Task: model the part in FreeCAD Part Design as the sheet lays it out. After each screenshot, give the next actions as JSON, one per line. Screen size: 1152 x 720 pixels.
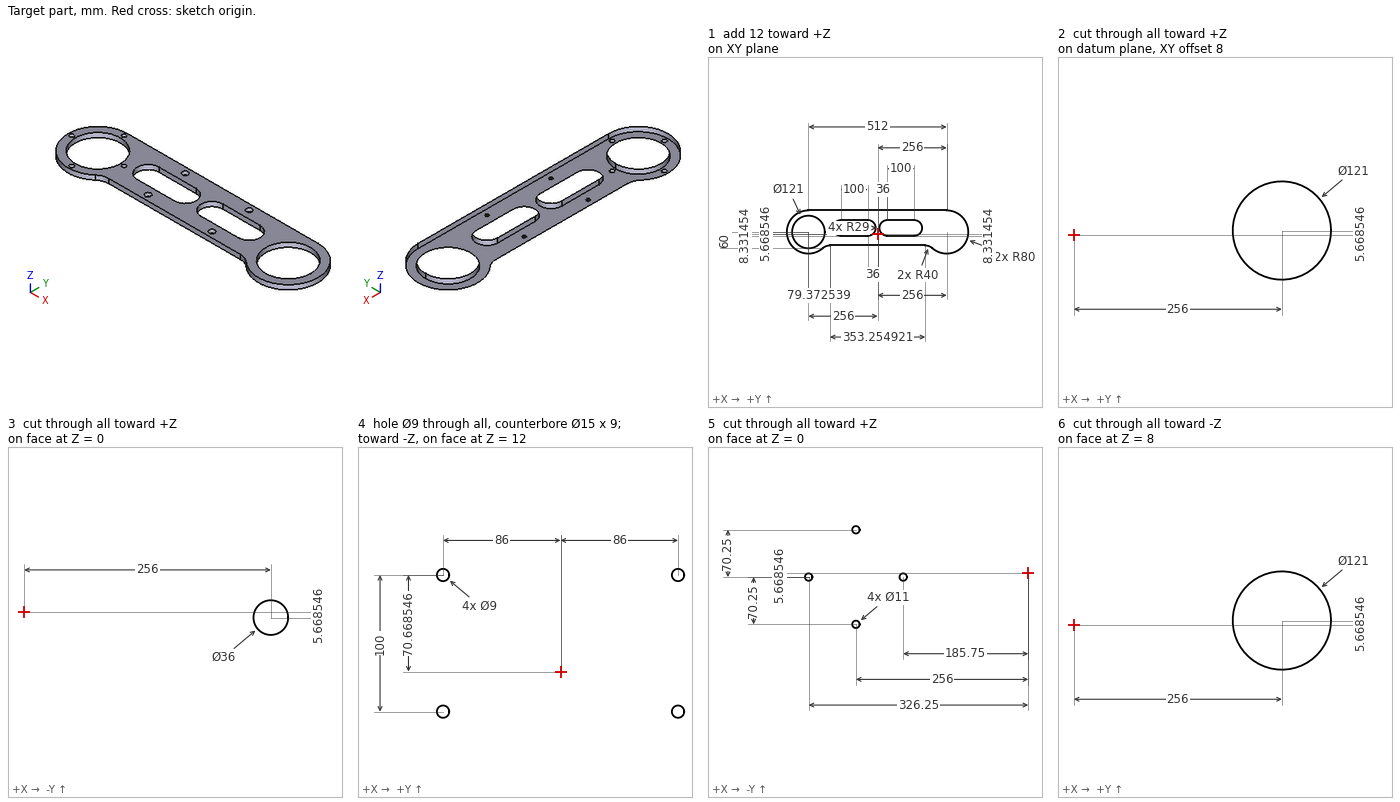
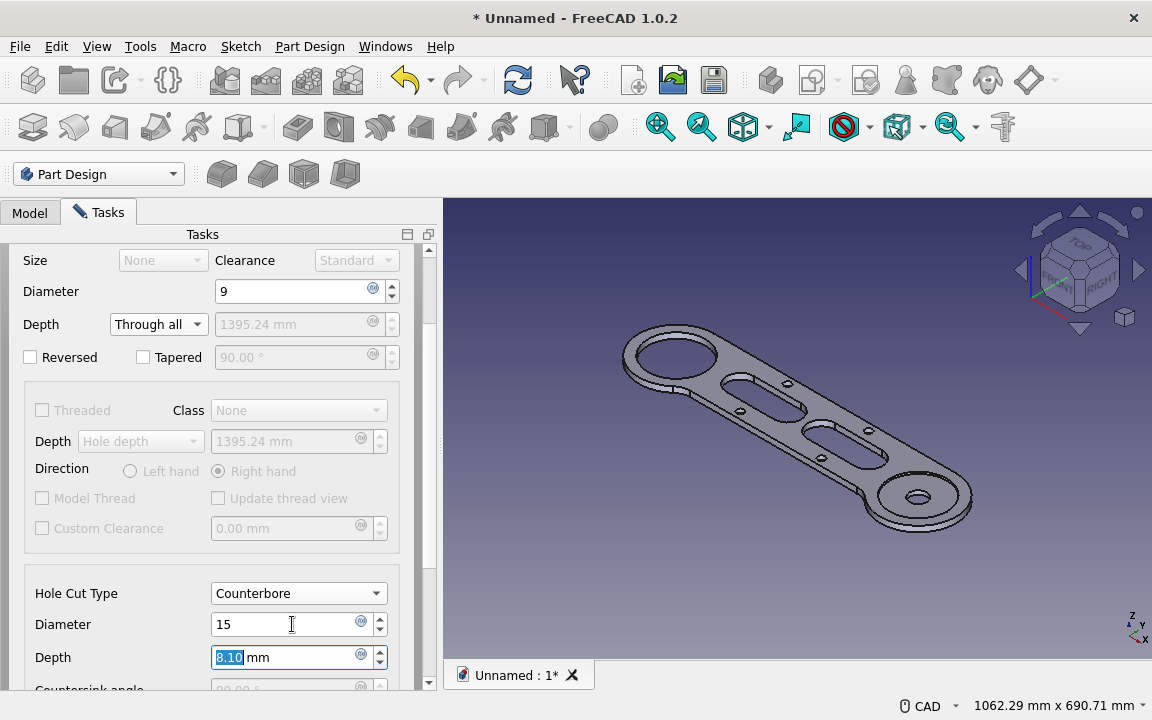
{"action": "type", "text": "9"}
{"action": "key", "text": "Tab"}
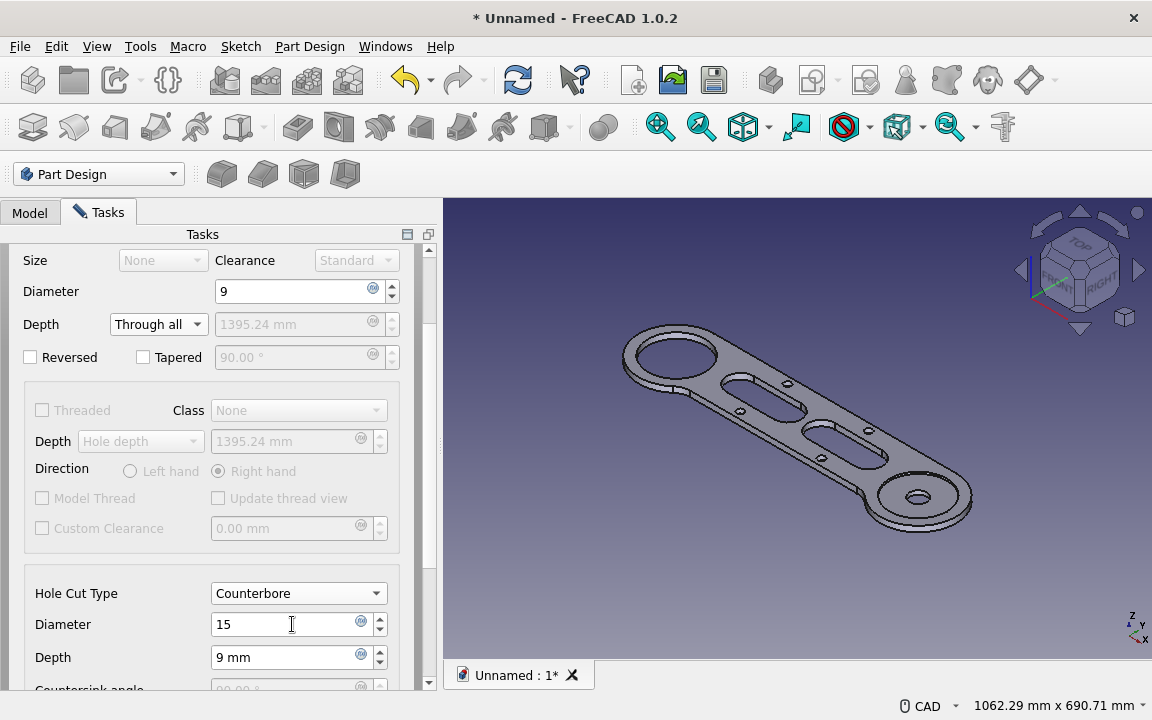
{"action": "scroll", "coordinate": [429, 467], "scroll_direction": "up", "scroll_amount": 3}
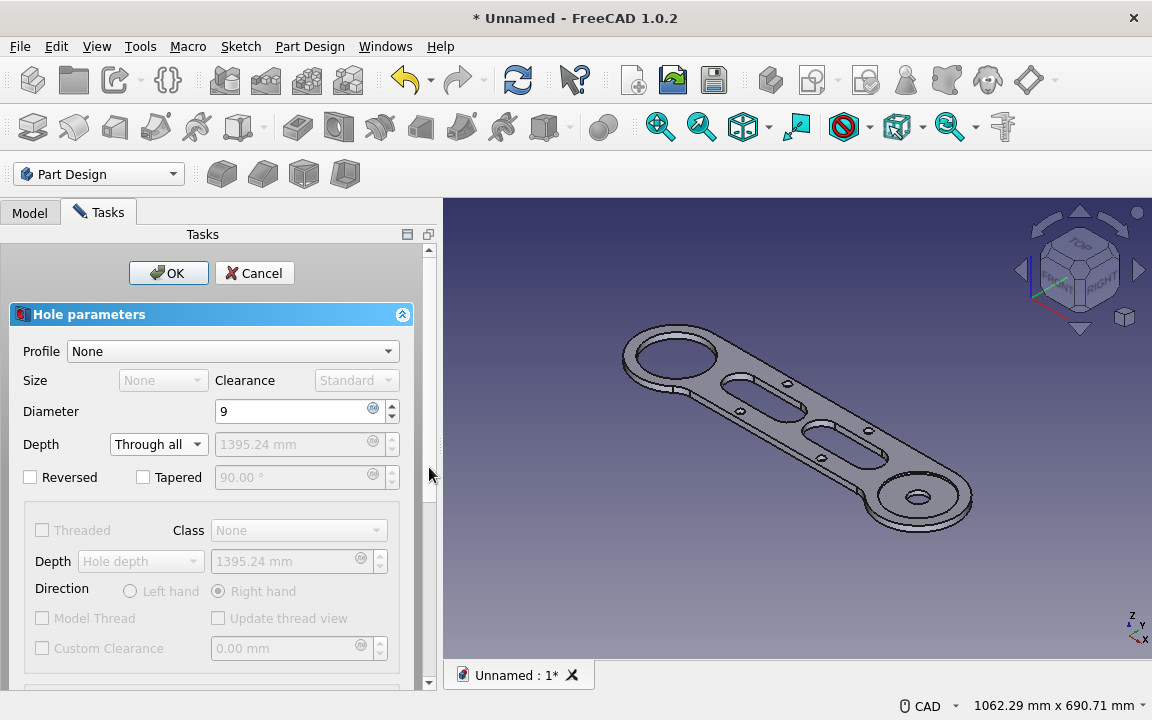
{"action": "left_click", "coordinate": [169, 273]}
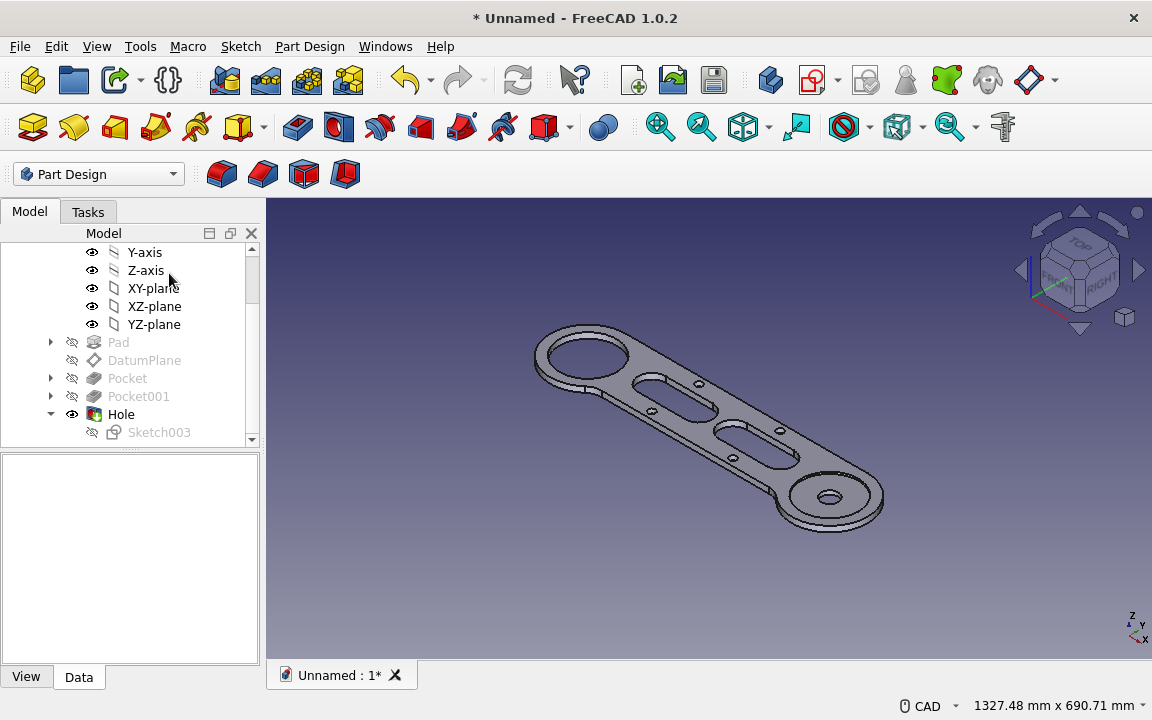
{"action": "key", "text": "5"}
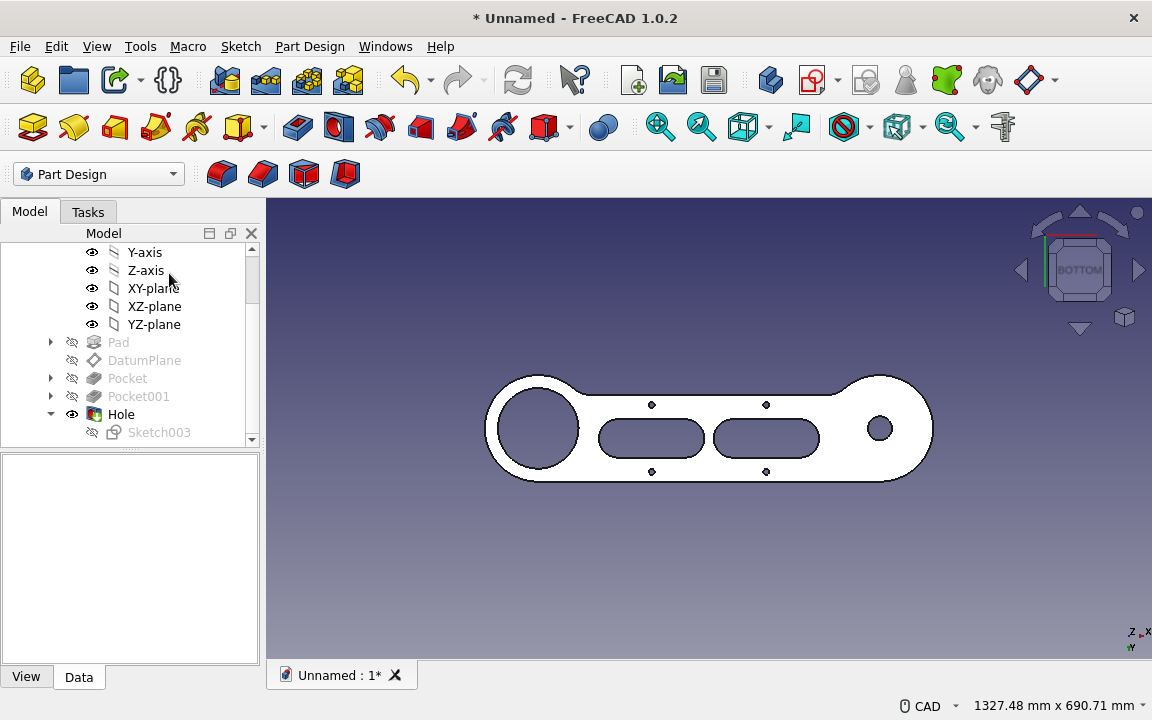
{"action": "left_click", "coordinate": [837, 458]}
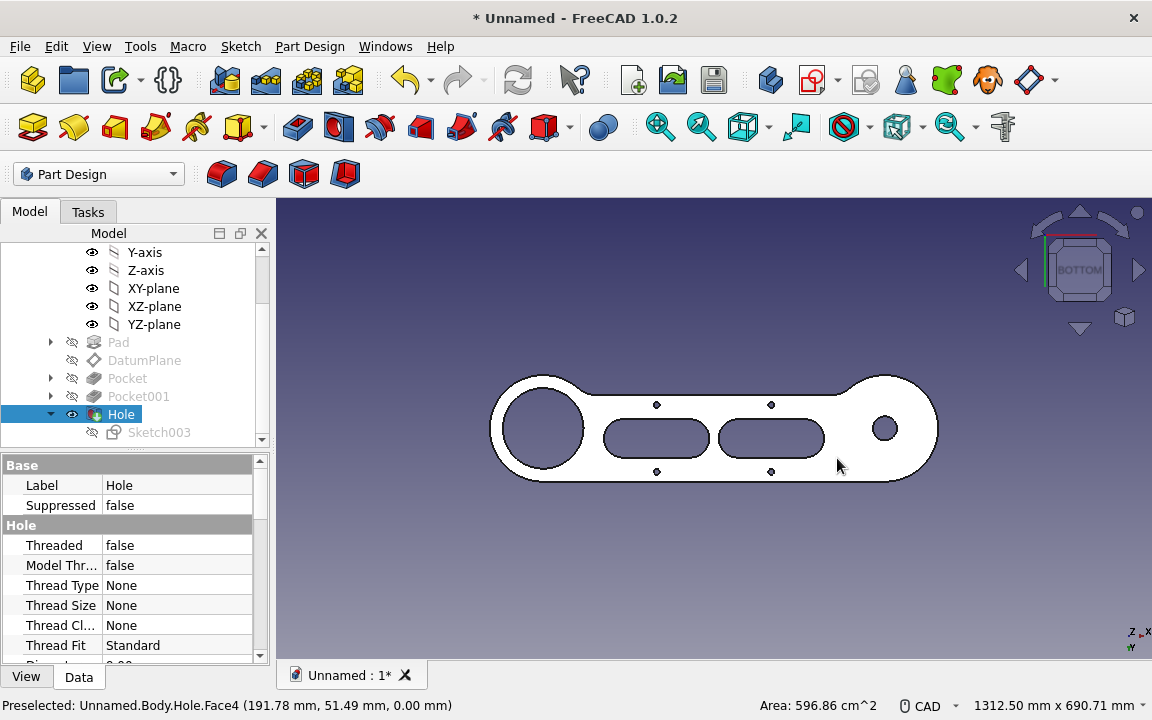
{"action": "left_click", "coordinate": [812, 80]}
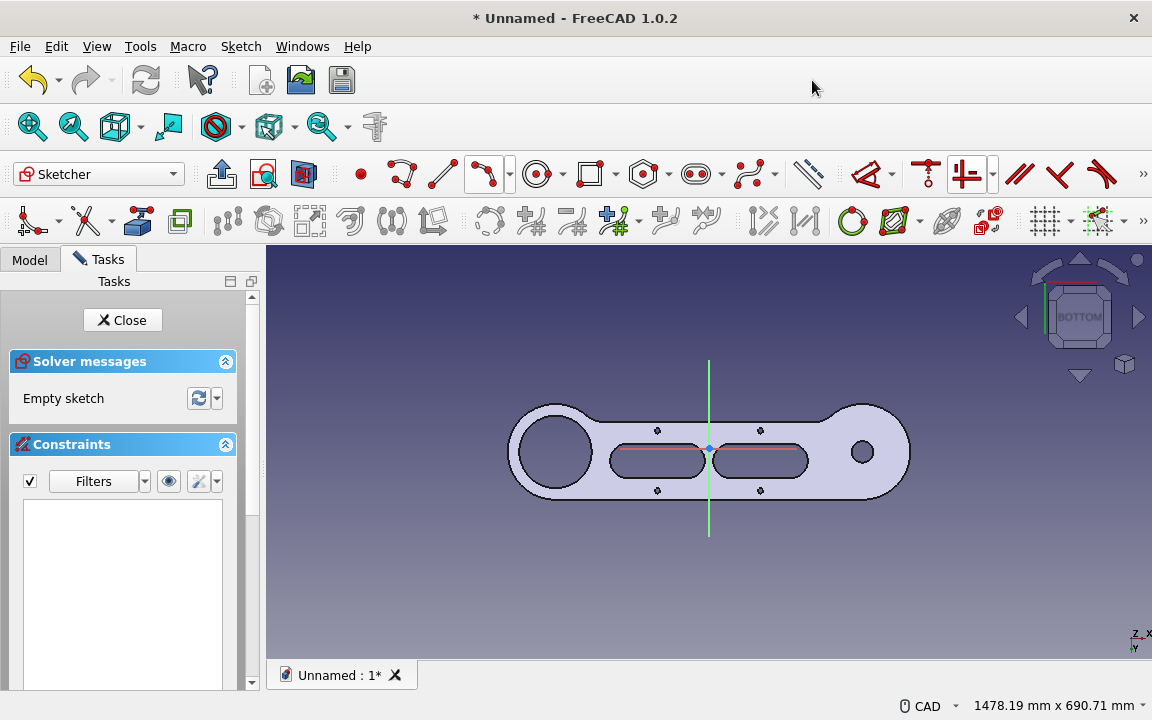
{"action": "scroll", "coordinate": [592, 452], "scroll_direction": "up", "scroll_amount": 5}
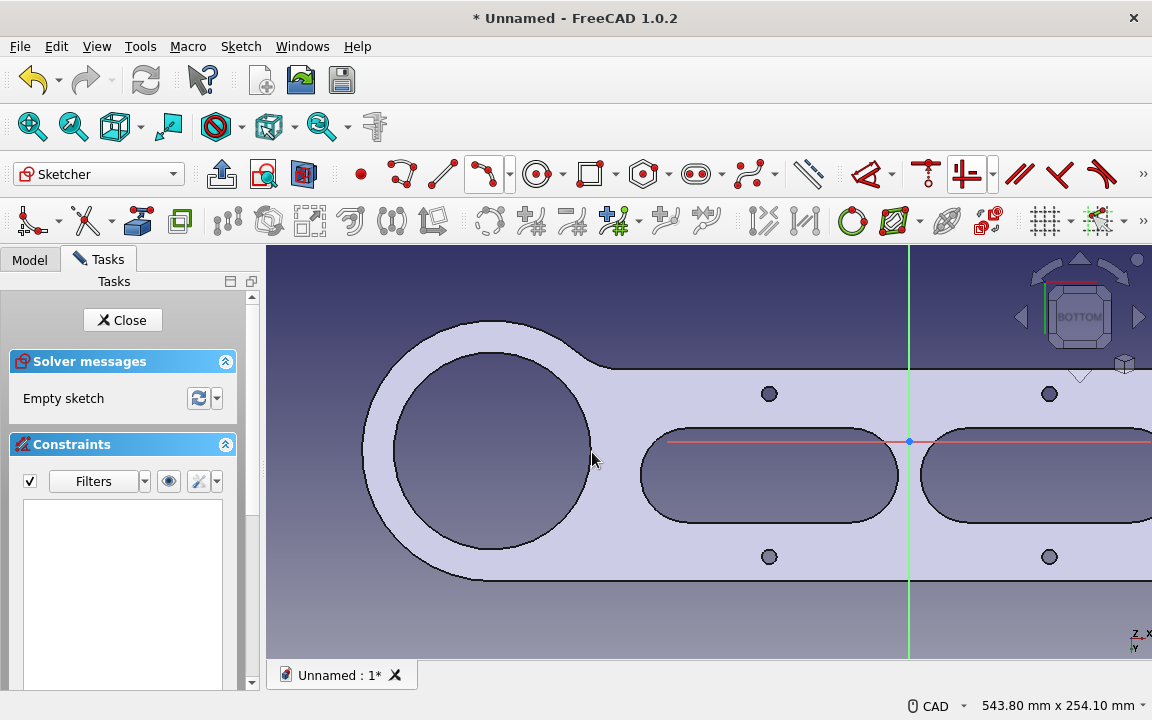
{"action": "left_click", "coordinate": [536, 174]}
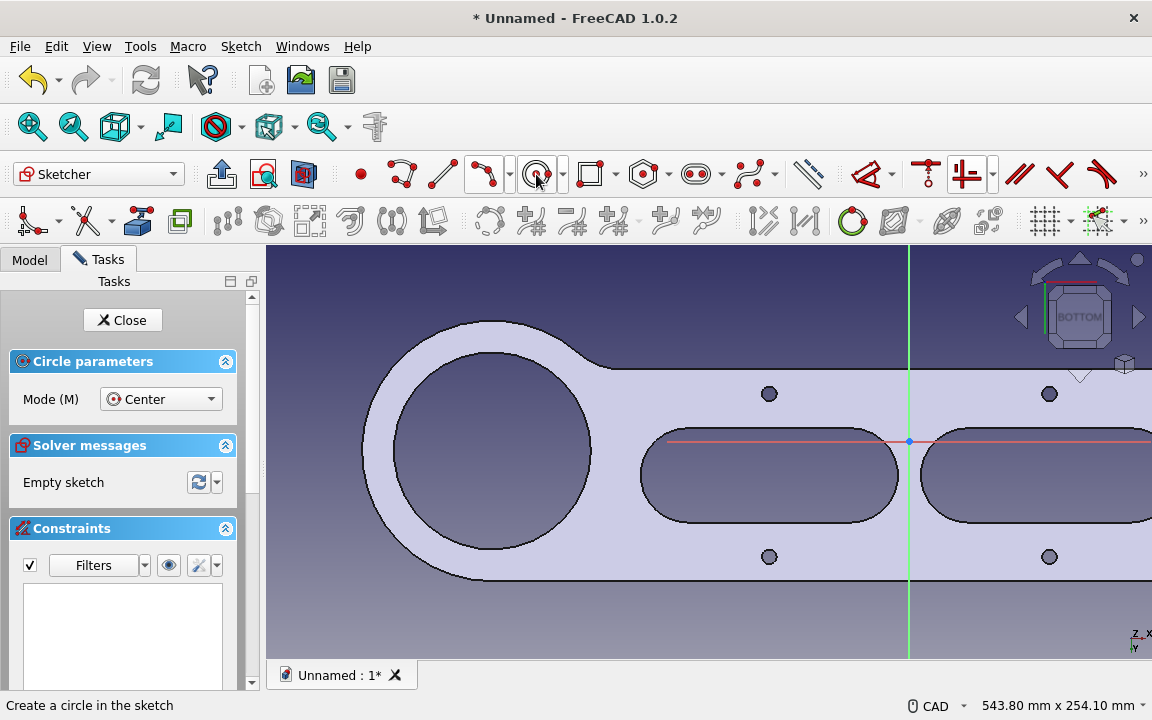
{"action": "scroll", "coordinate": [492, 565], "scroll_direction": "up", "scroll_amount": 5}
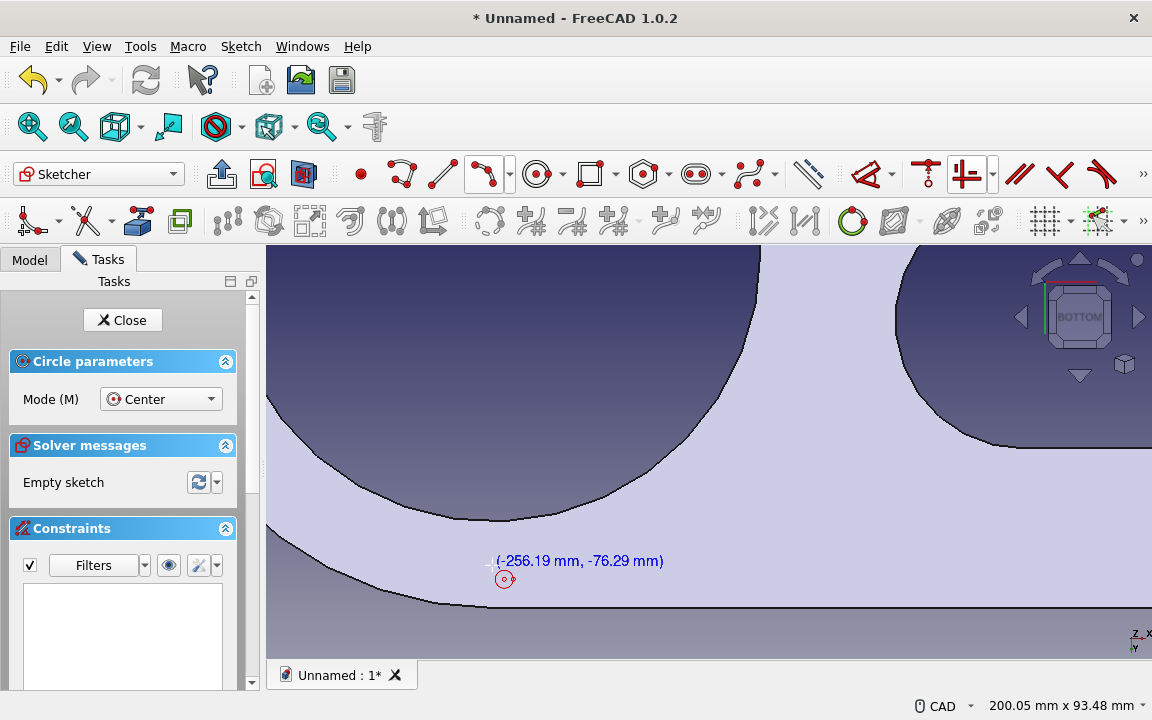
{"action": "left_click", "coordinate": [492, 565]}
{"action": "mouse_move", "coordinate": [510, 548]}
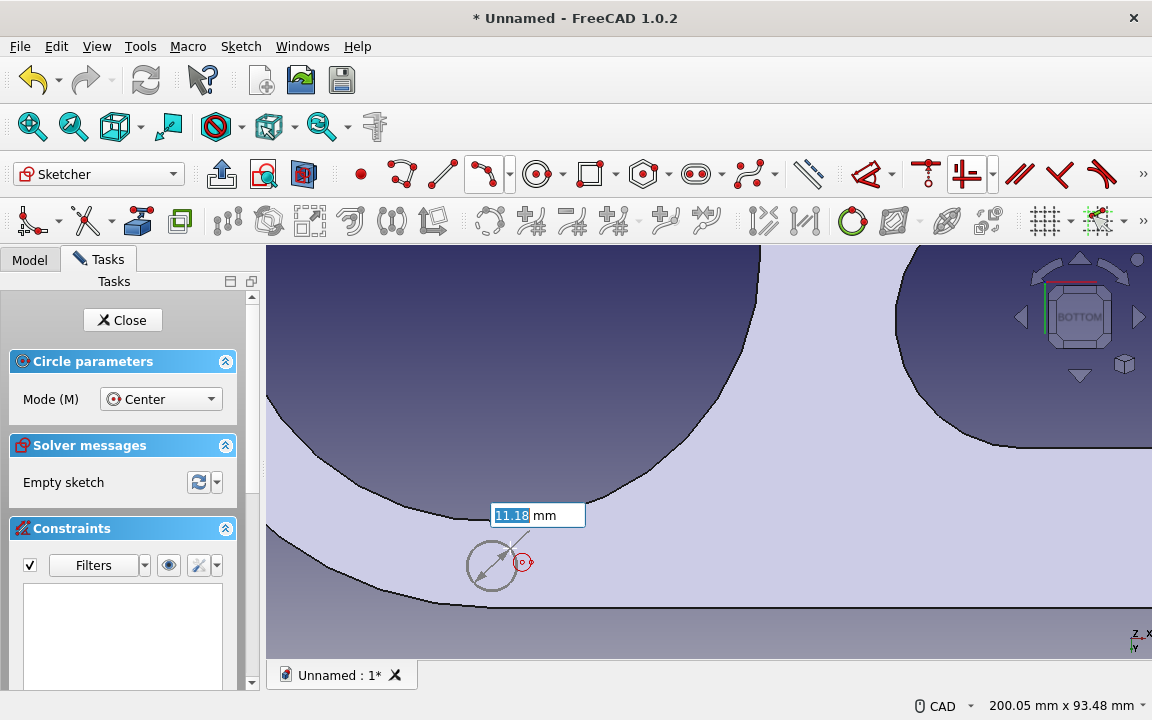
{"action": "type", "text": "11"}
{"action": "key", "text": "Return"}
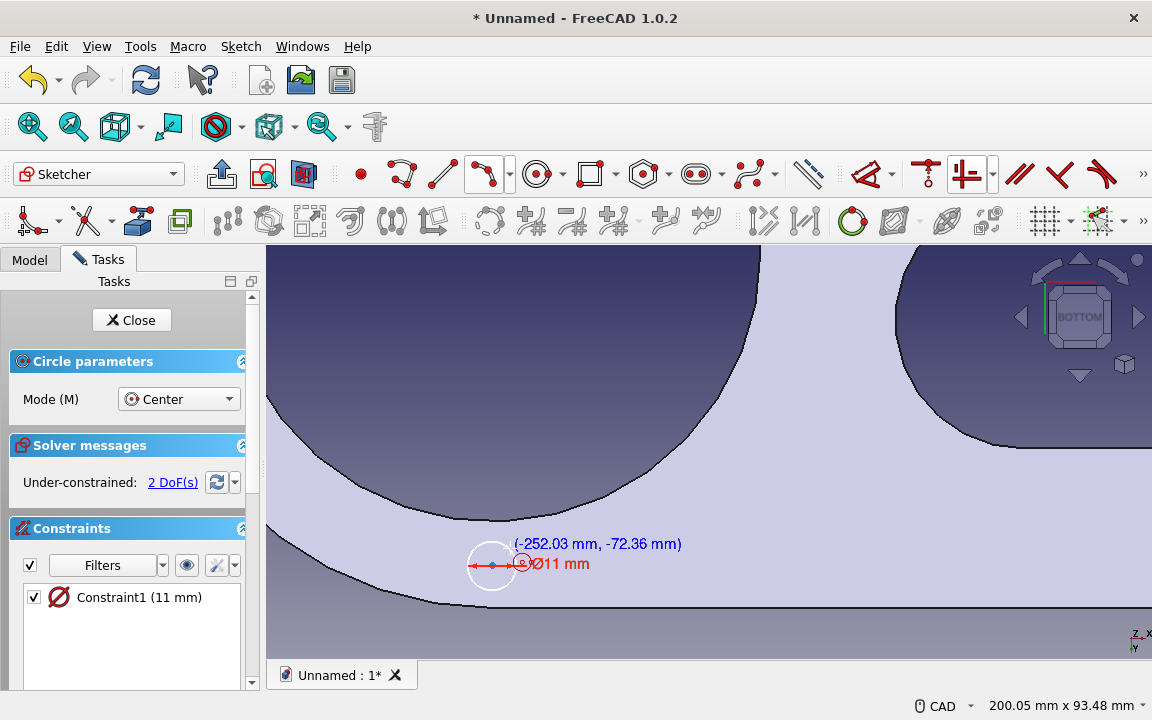
{"action": "scroll", "coordinate": [494, 567], "scroll_direction": "down", "scroll_amount": 5}